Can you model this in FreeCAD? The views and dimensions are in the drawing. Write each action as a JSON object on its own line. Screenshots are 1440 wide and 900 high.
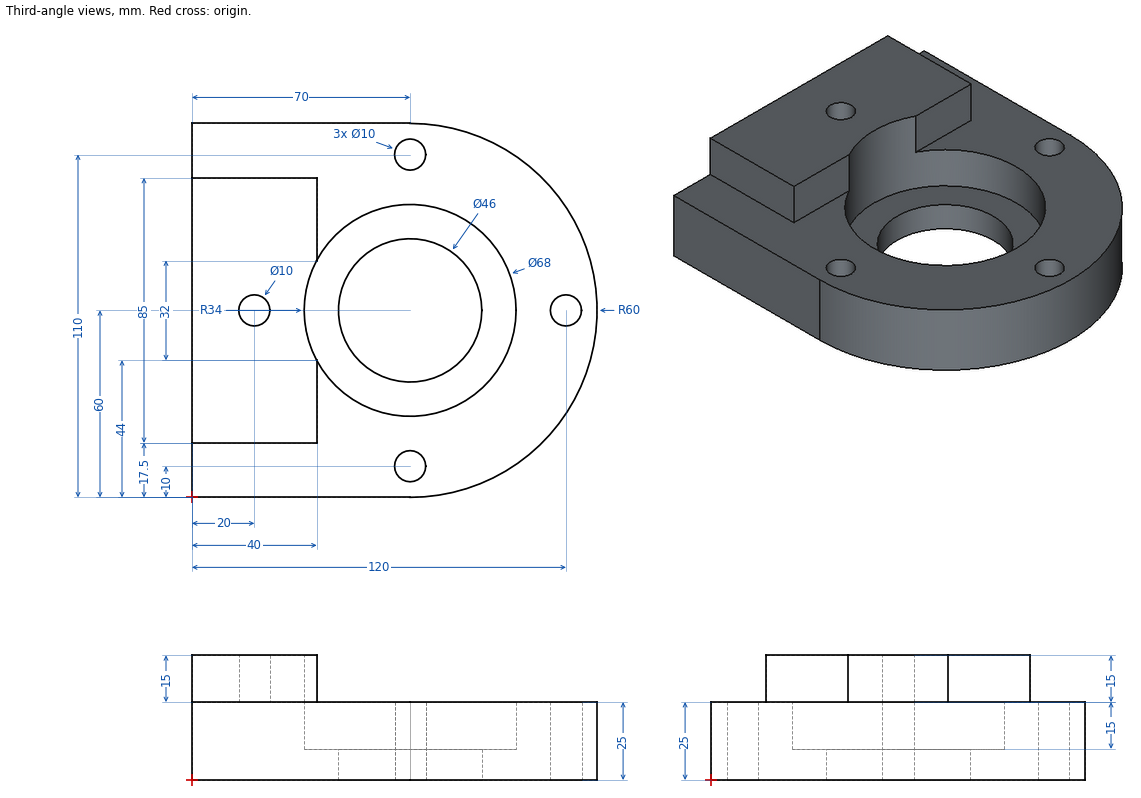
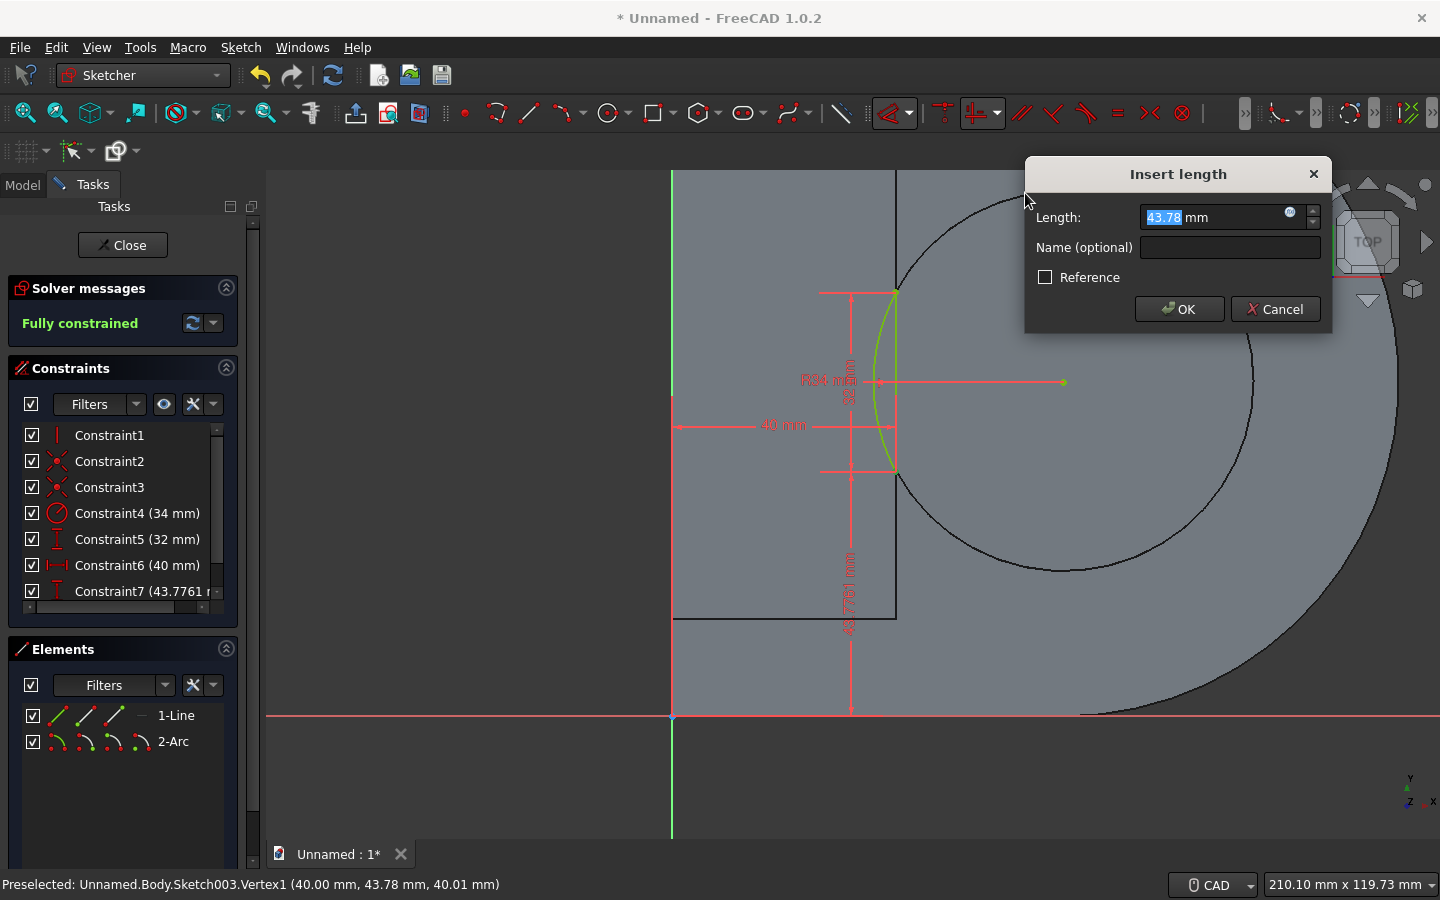
{"action": "type", "text": "44"}
{"action": "key", "text": "Return"}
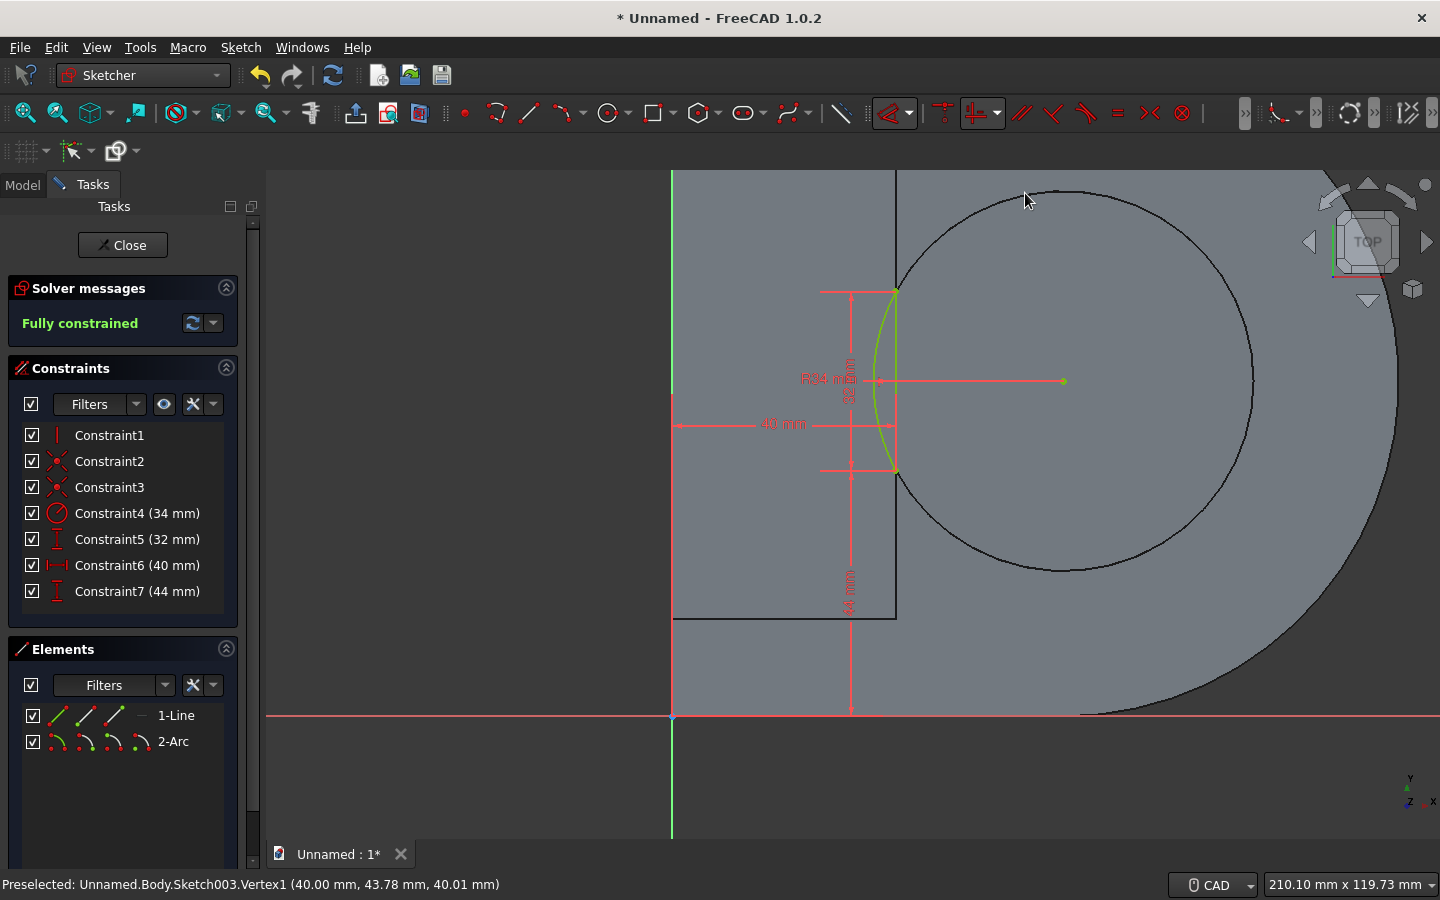
{"action": "left_click", "coordinate": [123, 245]}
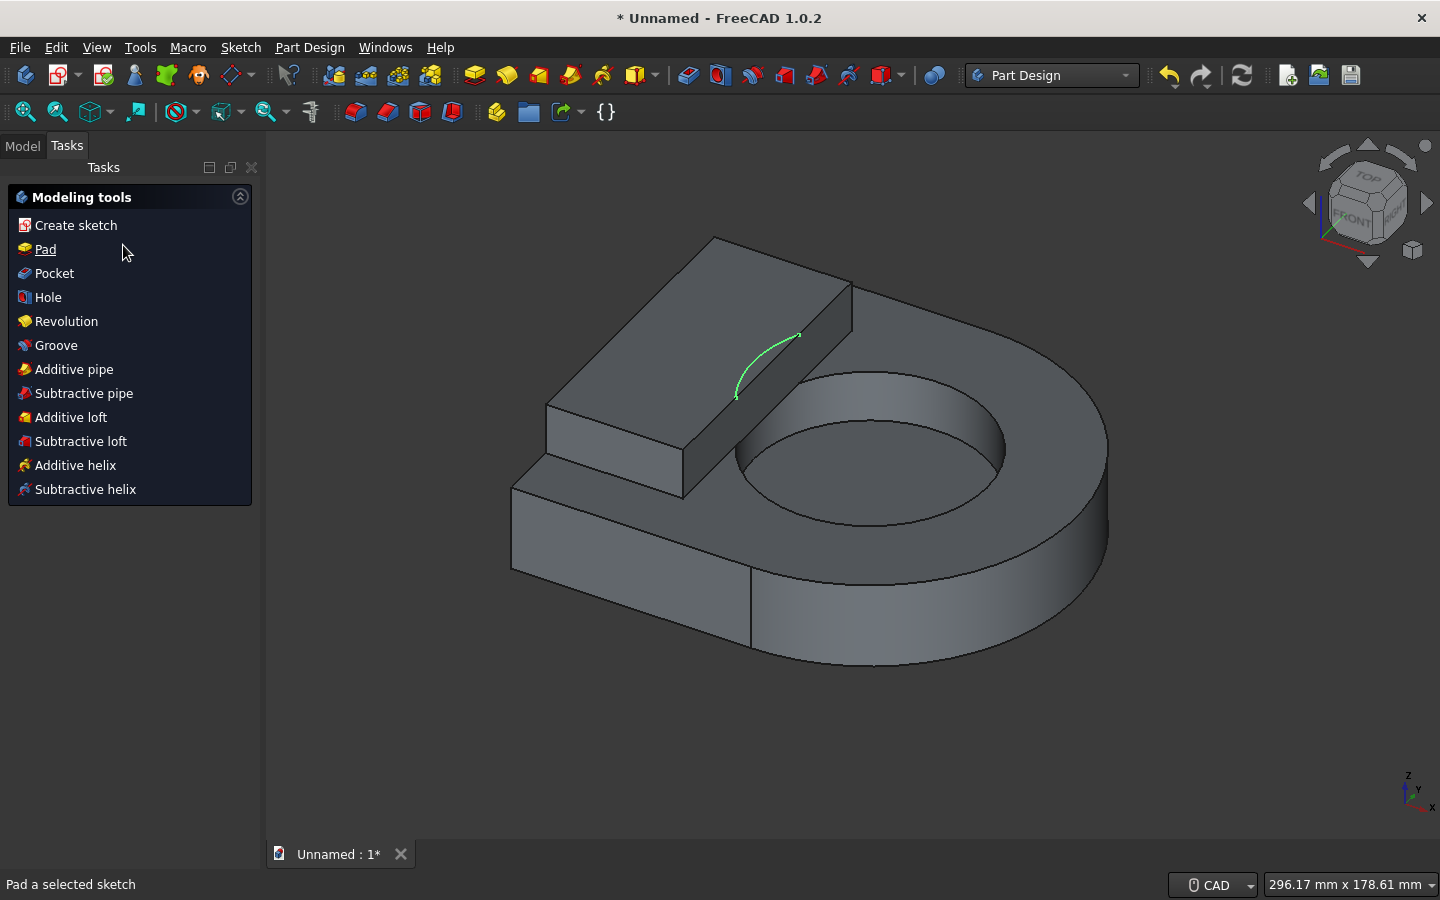
{"action": "left_click", "coordinate": [690, 76]}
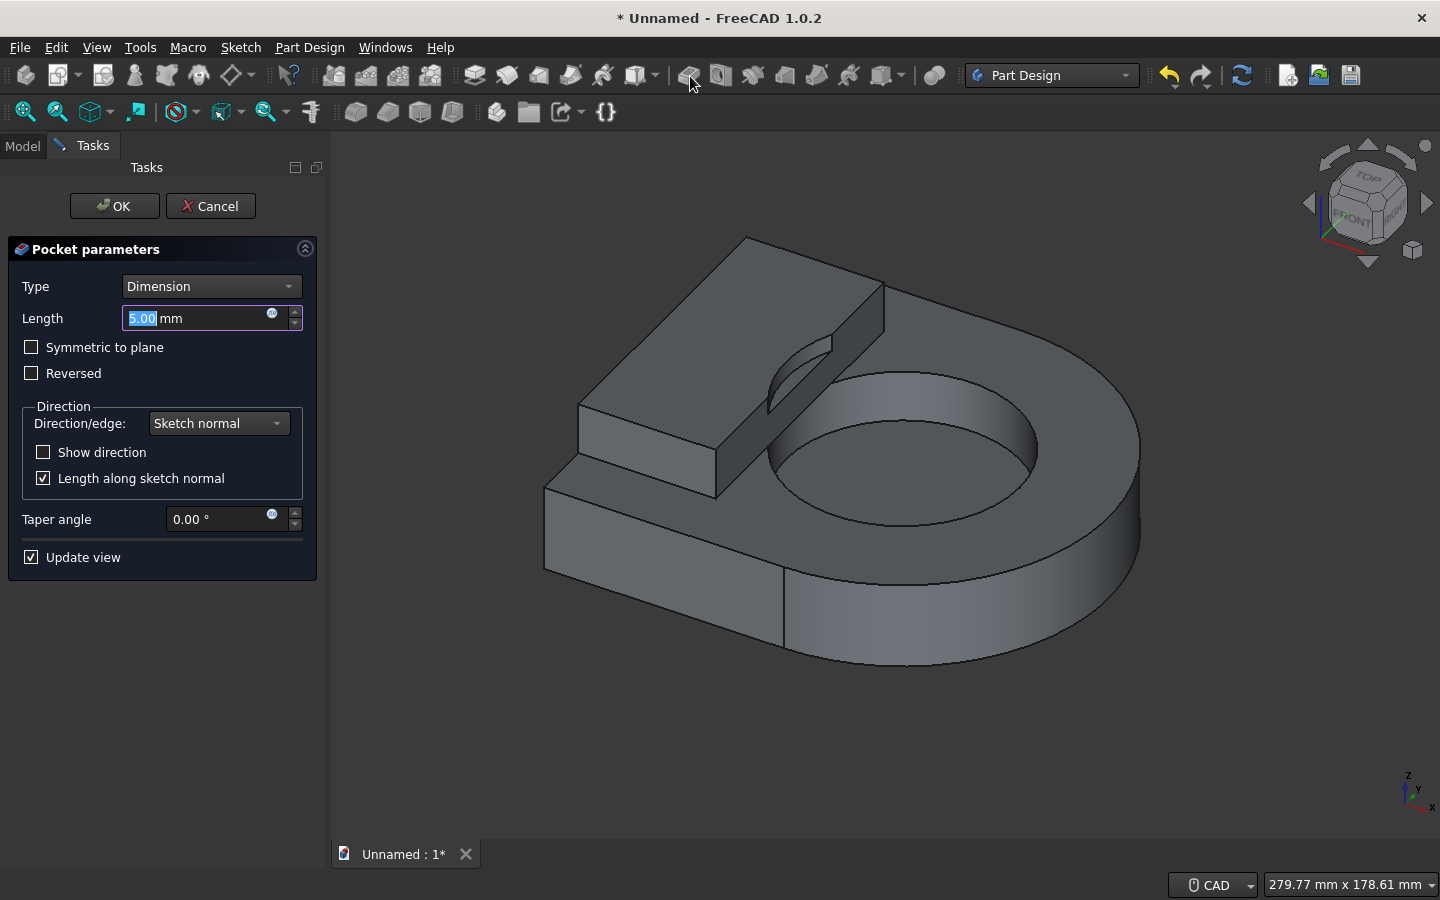
{"action": "type", "text": "15"}
{"action": "key", "text": "Tab"}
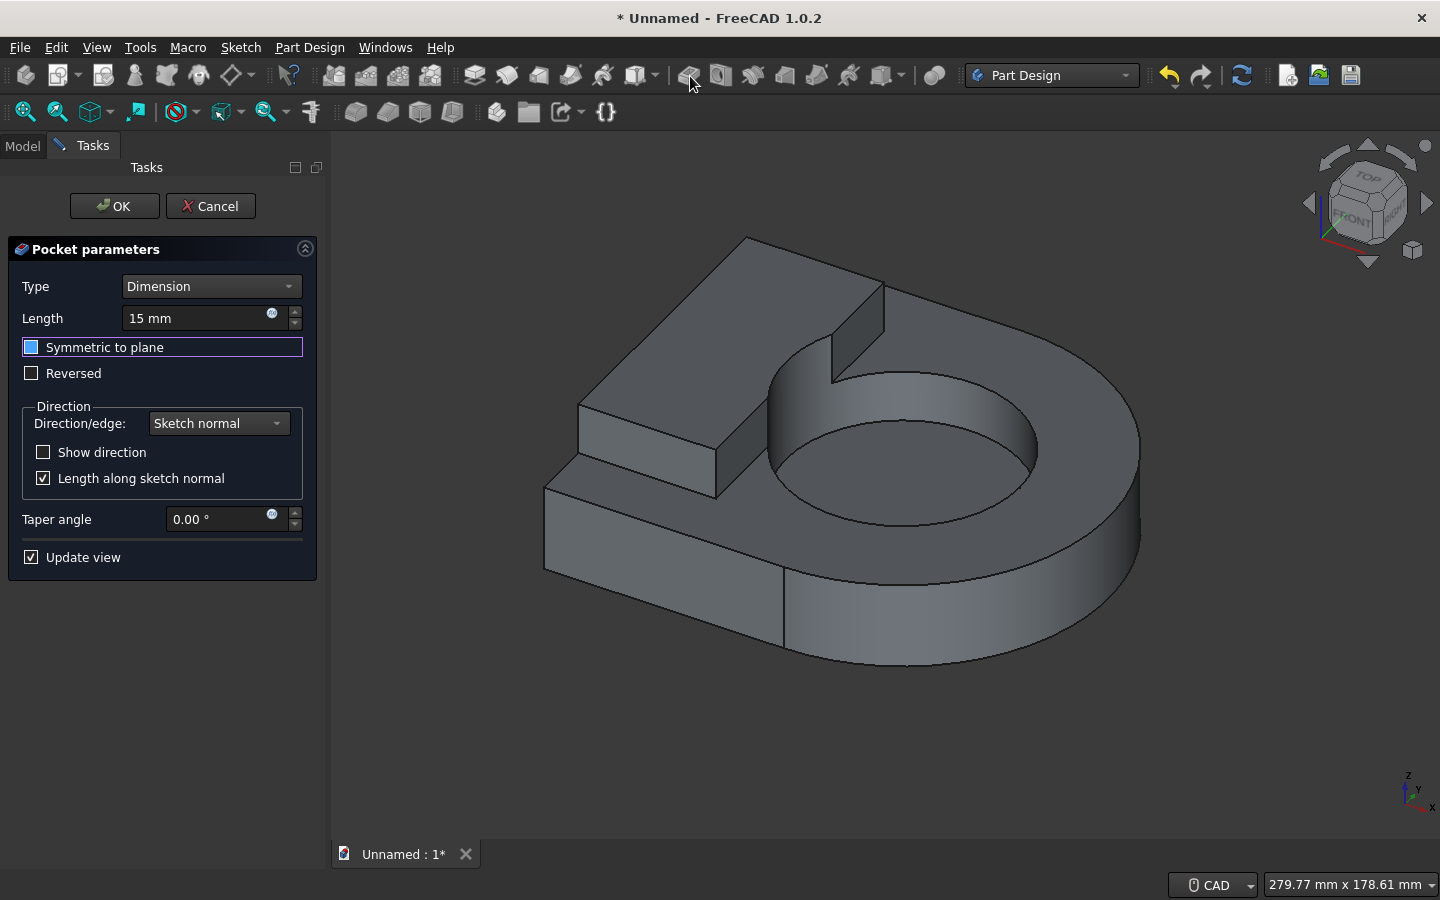
{"action": "left_click", "coordinate": [115, 206]}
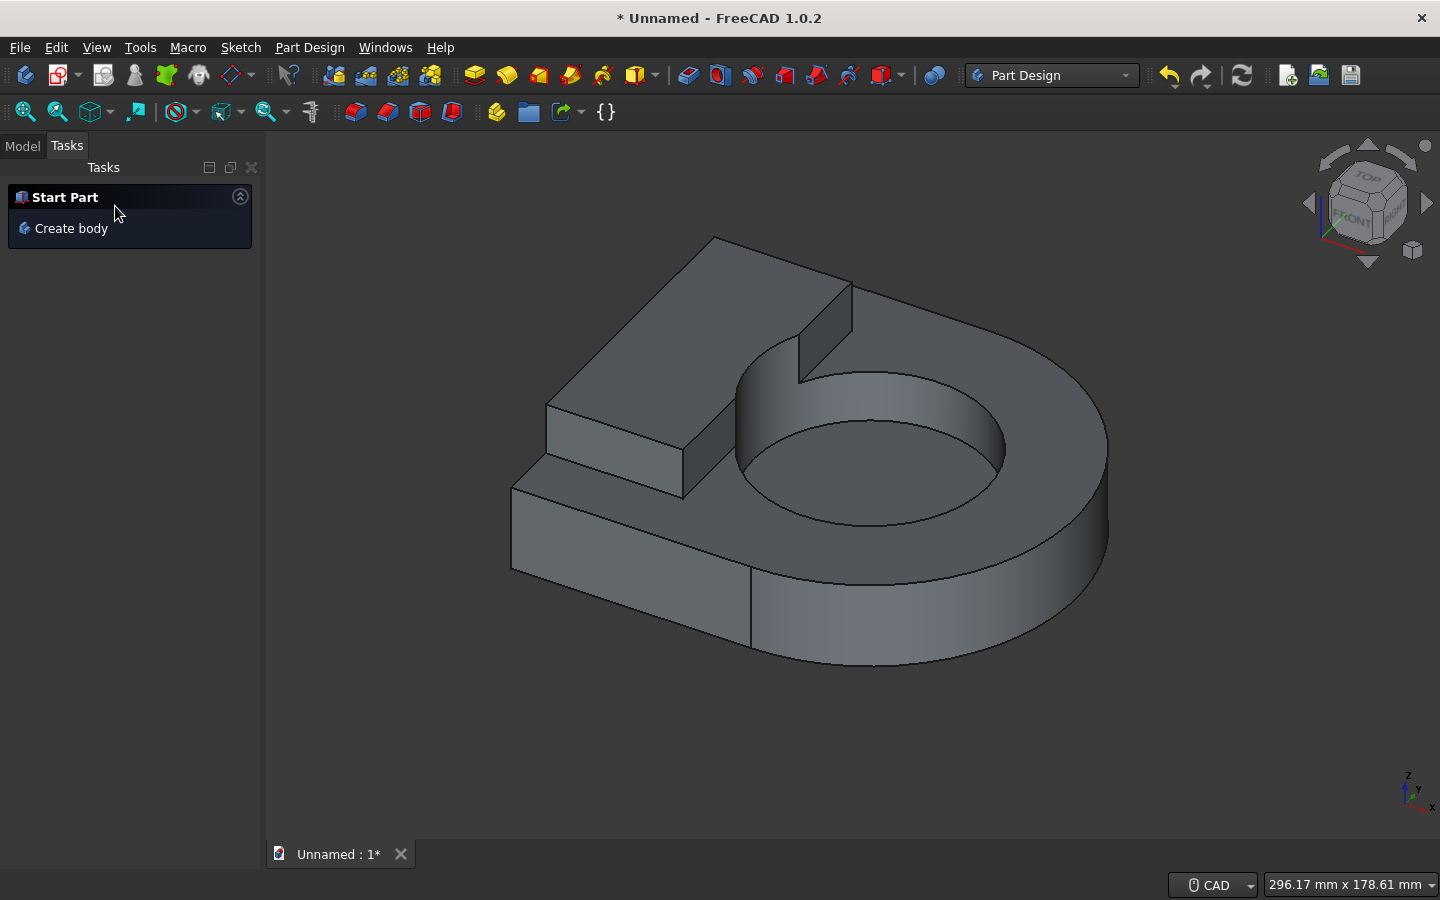
{"action": "left_click", "coordinate": [870, 497]}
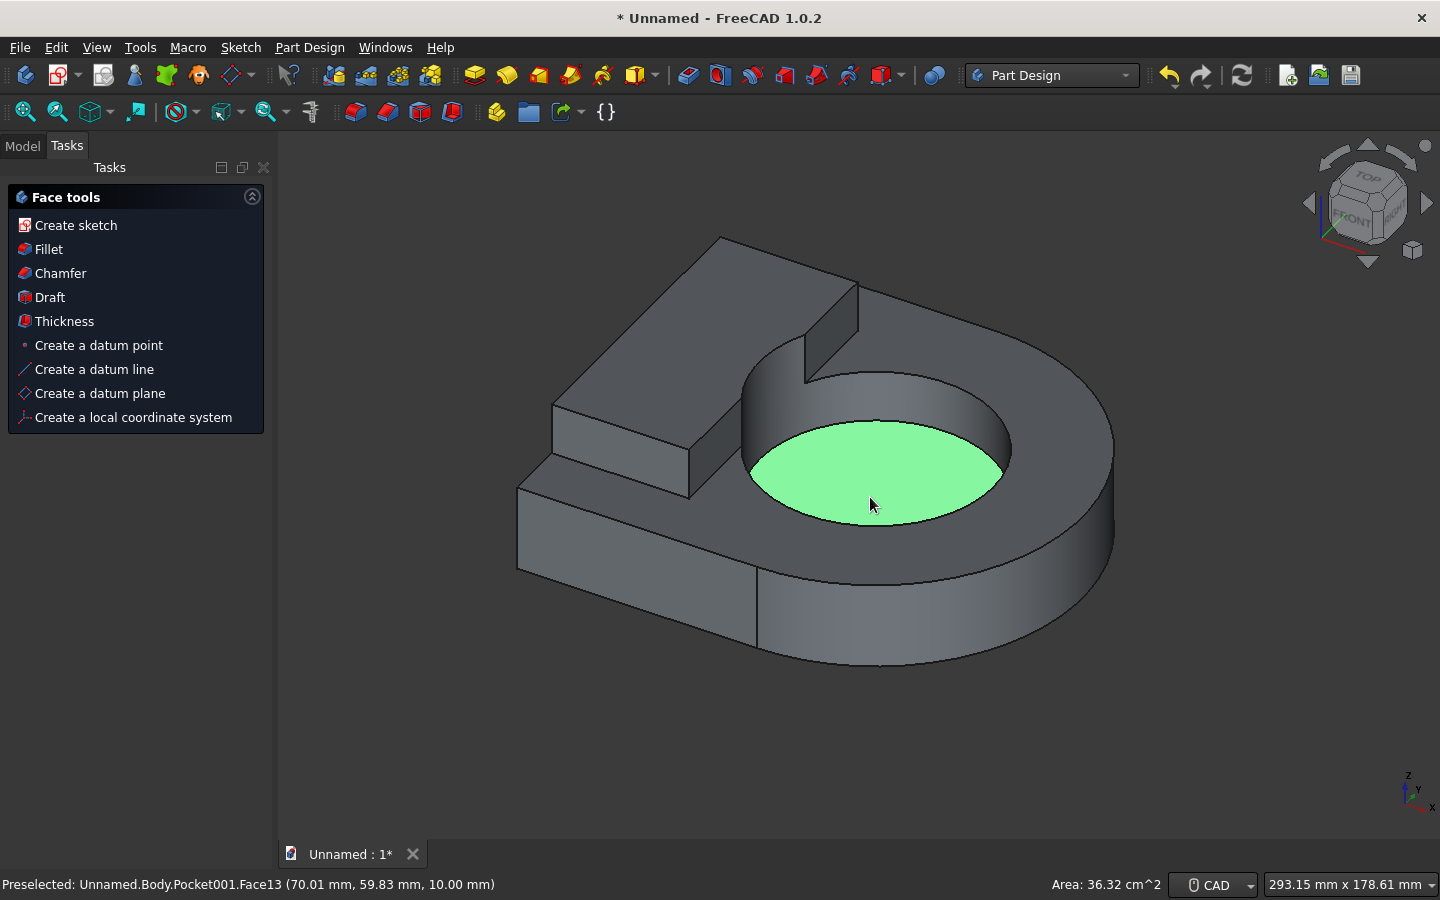
{"action": "left_click", "coordinate": [58, 76]}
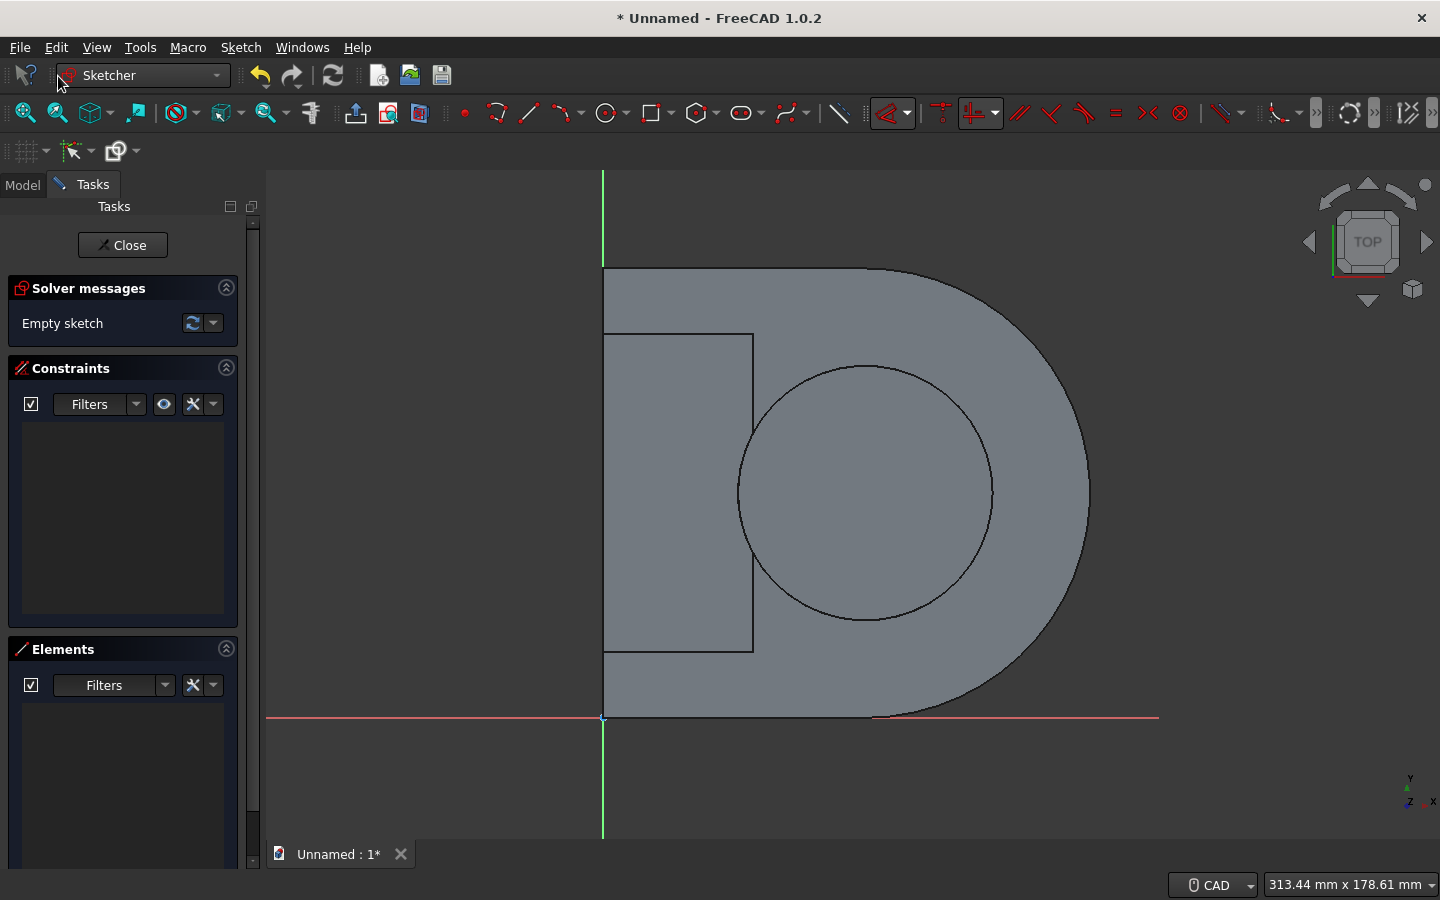
{"action": "scroll", "coordinate": [763, 680], "scroll_direction": "up", "scroll_amount": 2}